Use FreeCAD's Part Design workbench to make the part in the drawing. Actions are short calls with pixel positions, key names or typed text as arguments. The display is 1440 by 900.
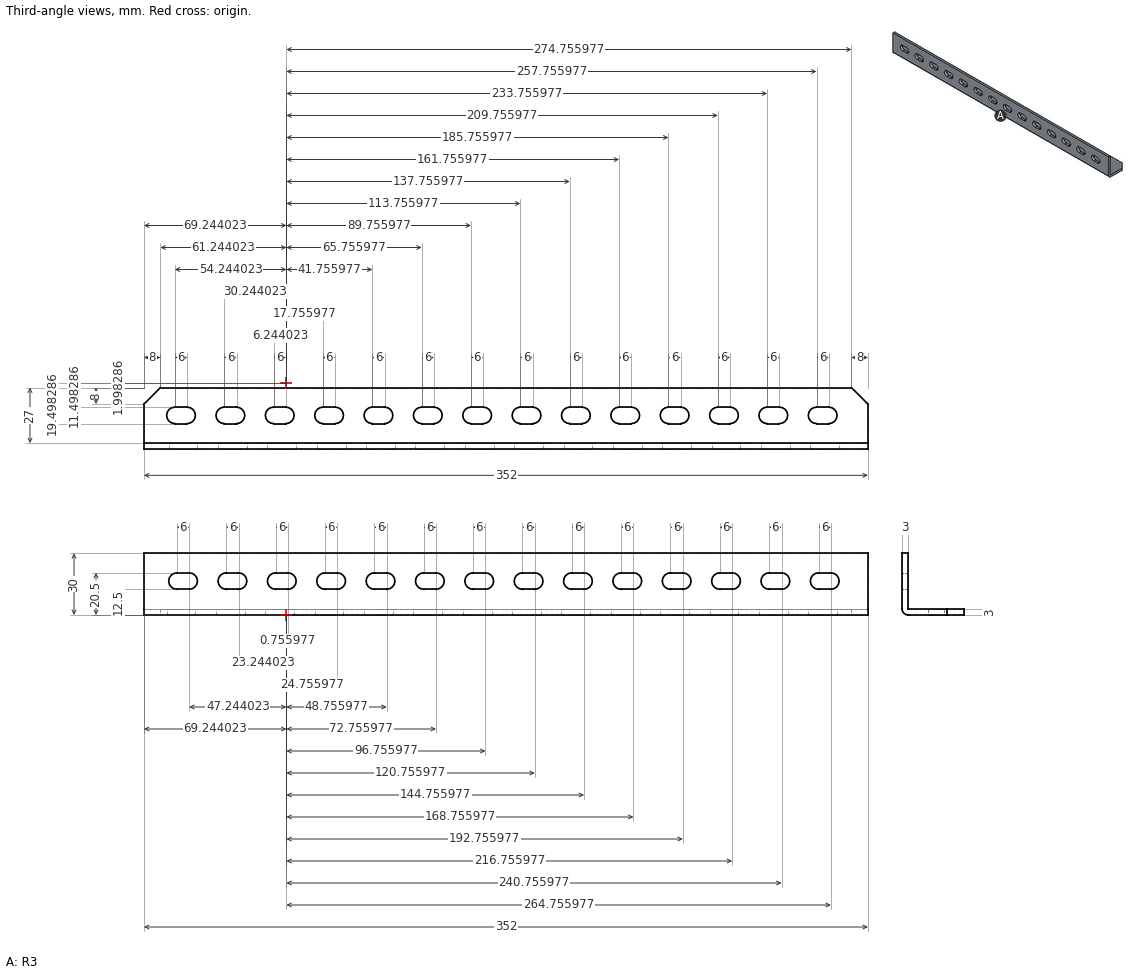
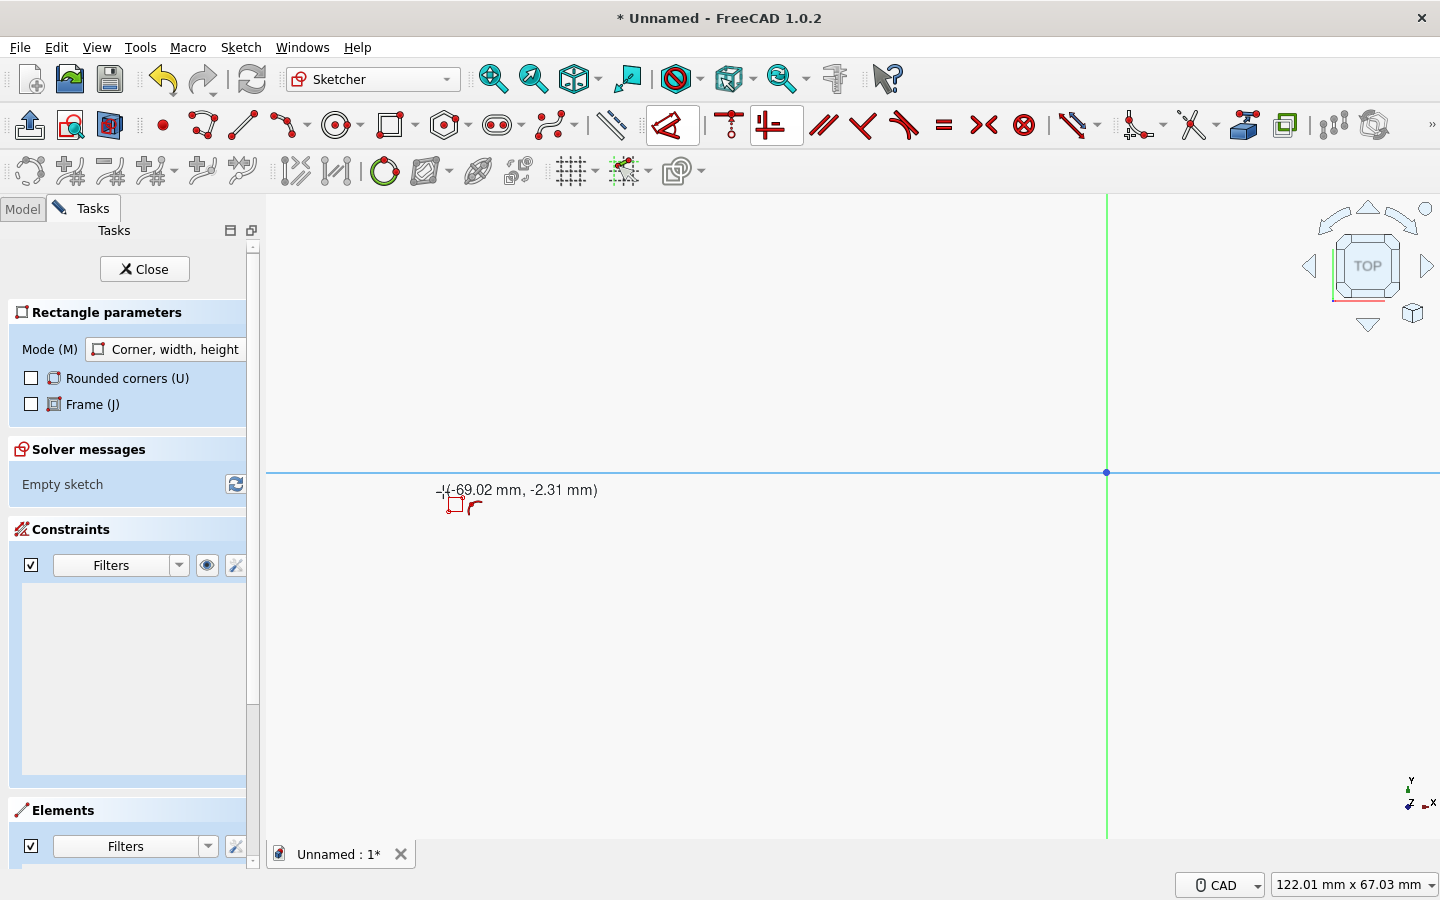
click(440, 492)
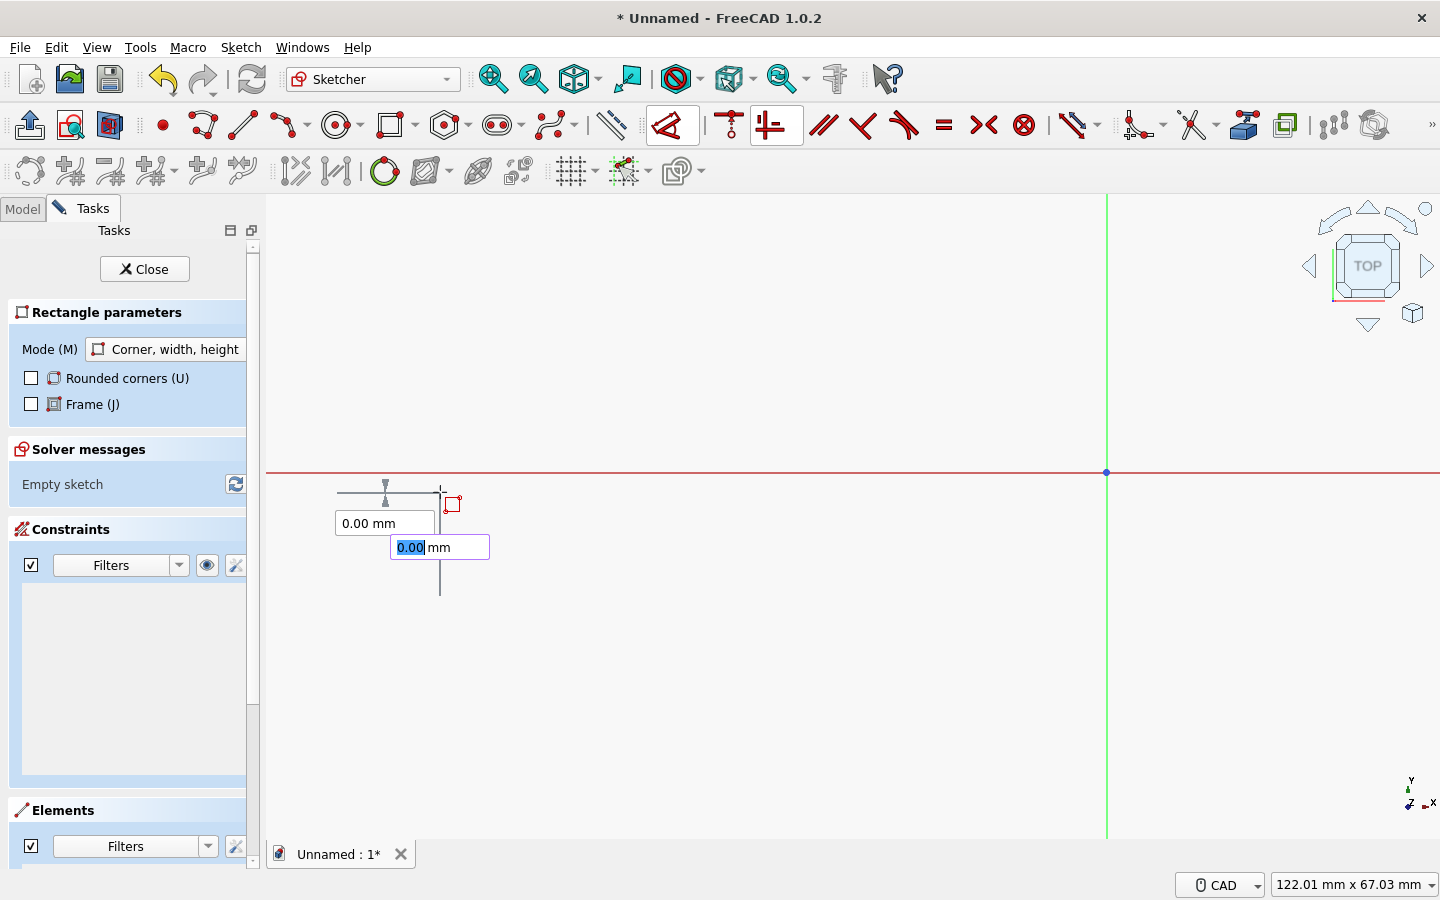
scroll(443, 492, down, 8)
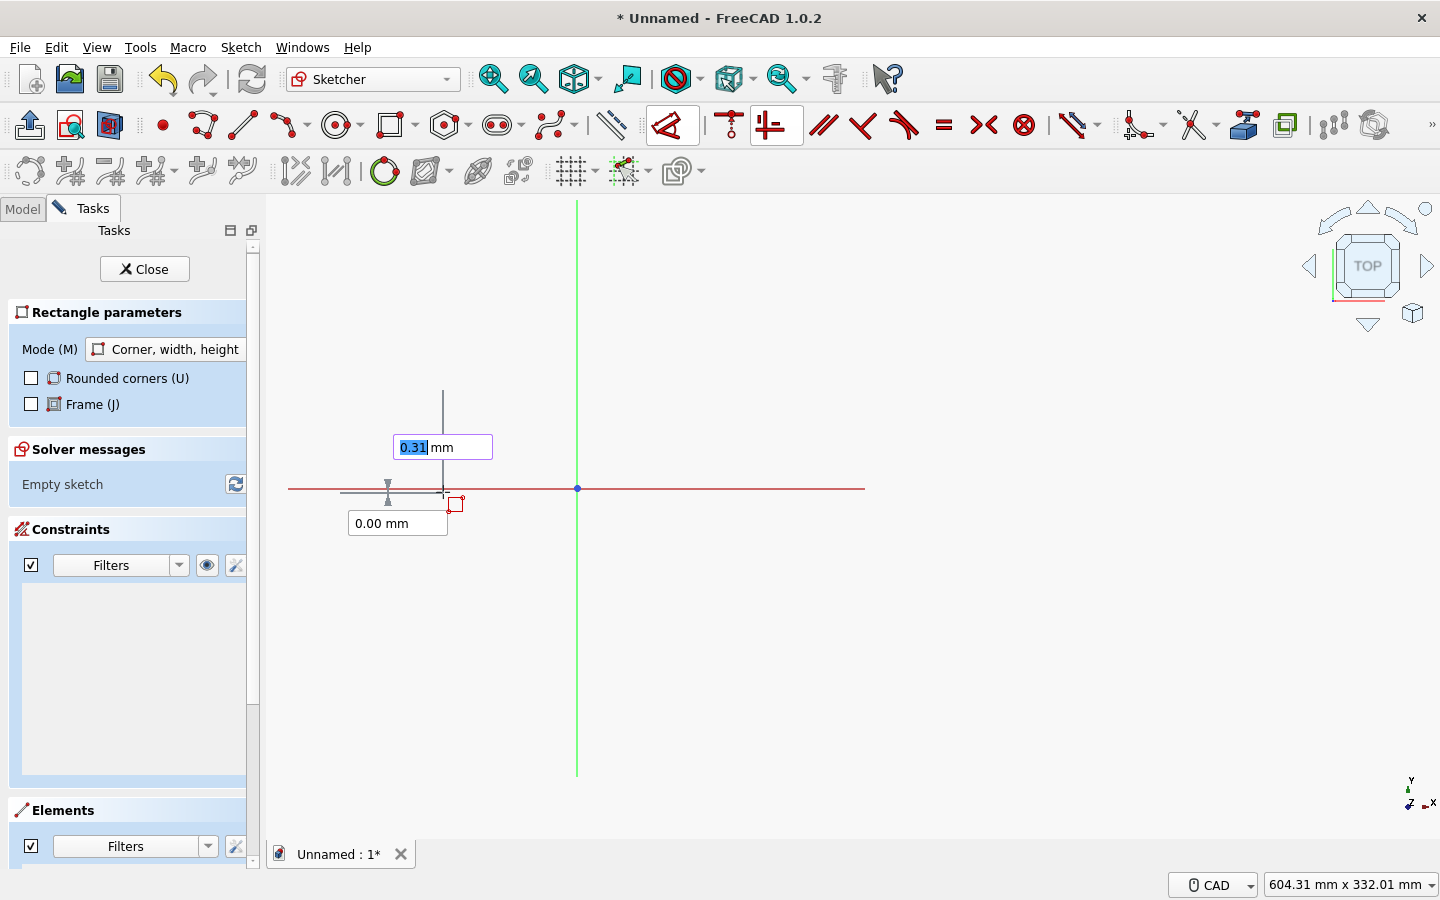
click(1126, 545)
key(Escape)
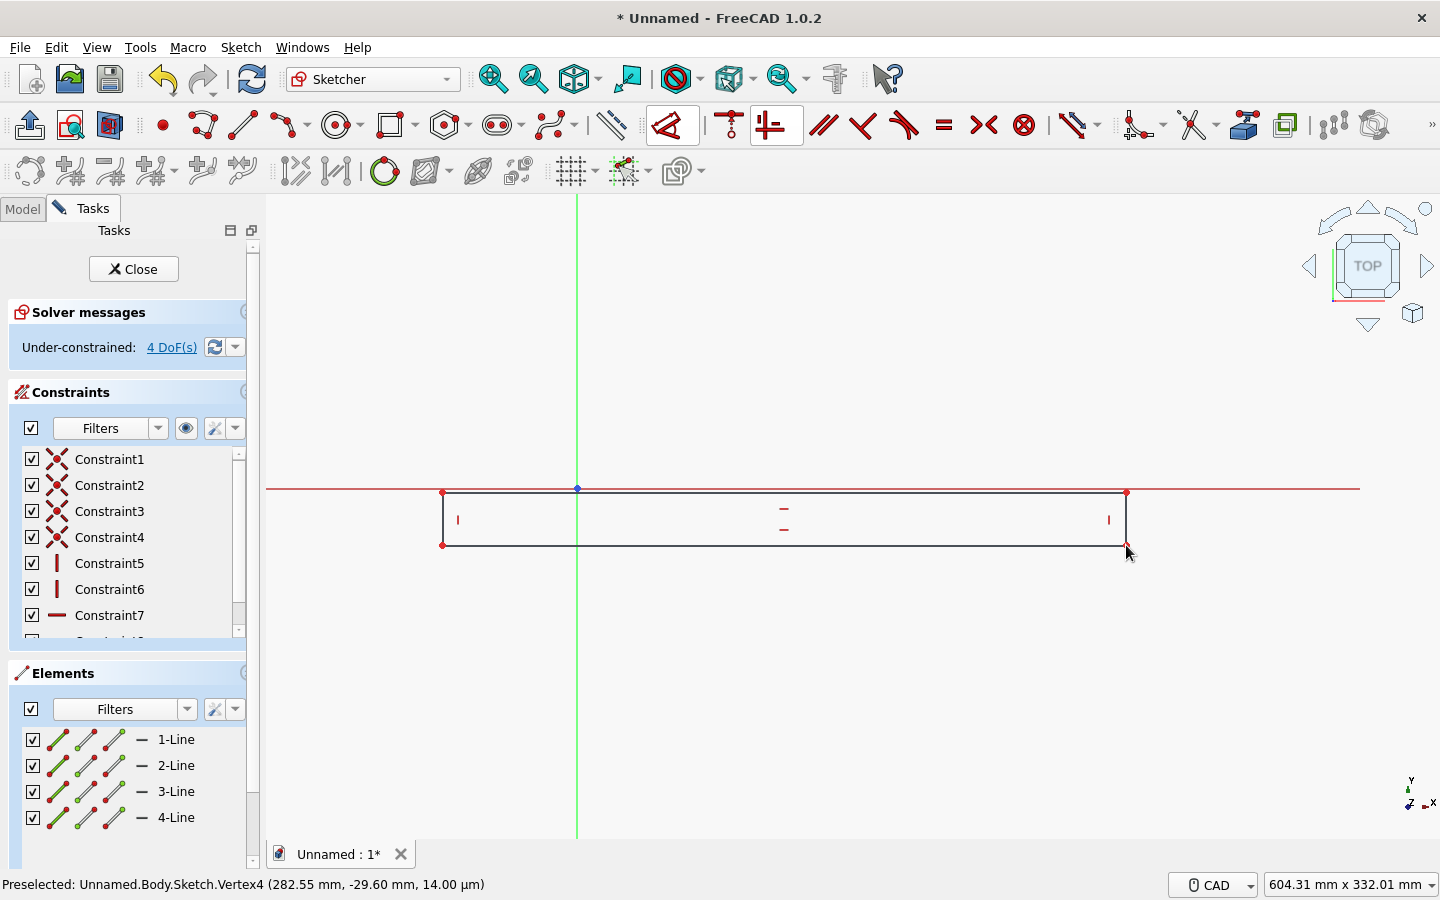
click(666, 126)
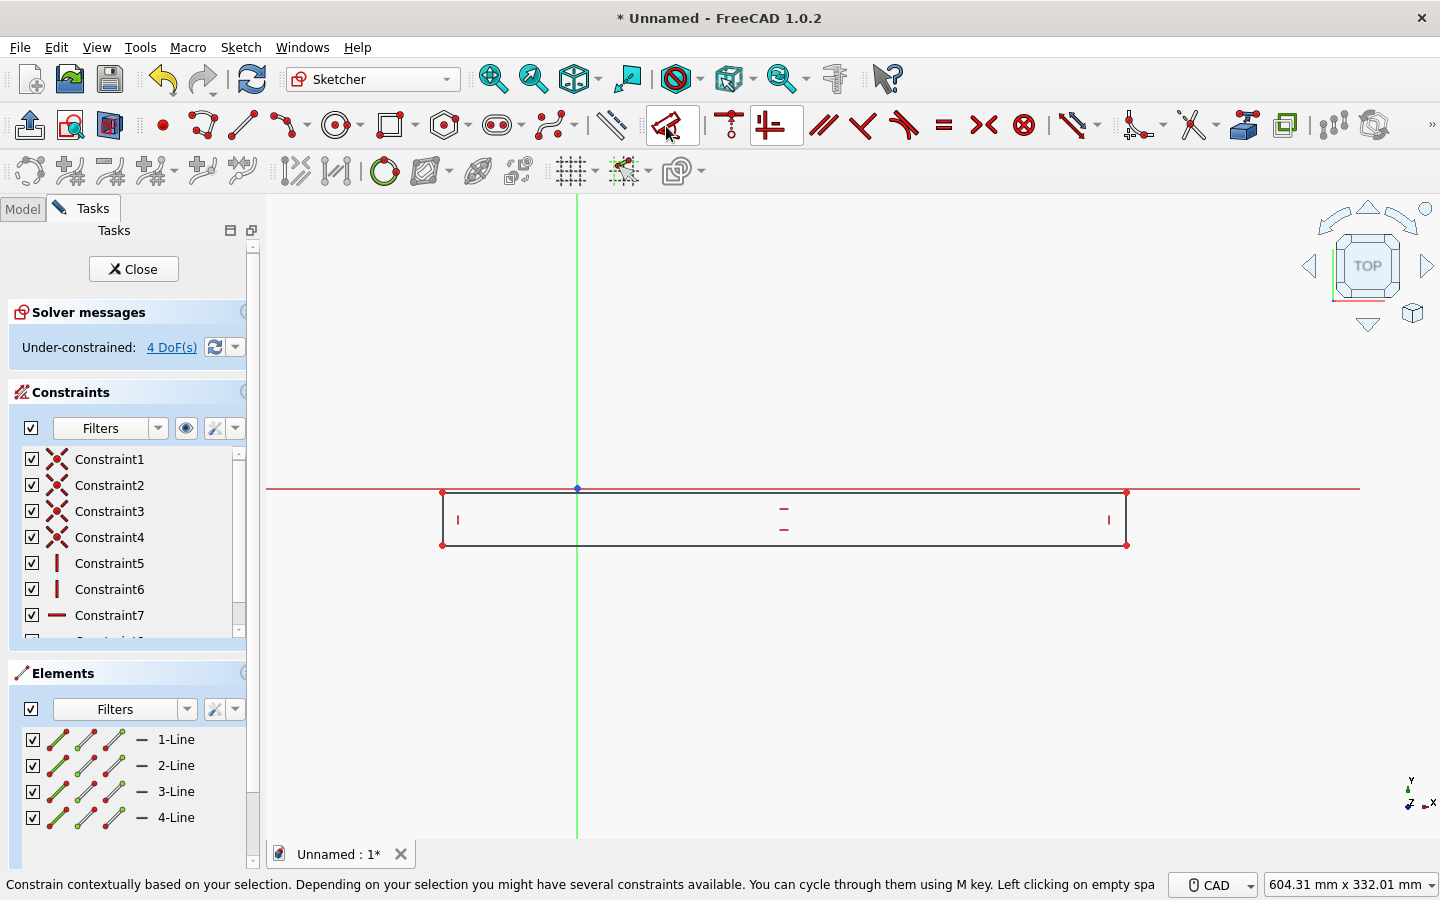
click(443, 509)
click(409, 519)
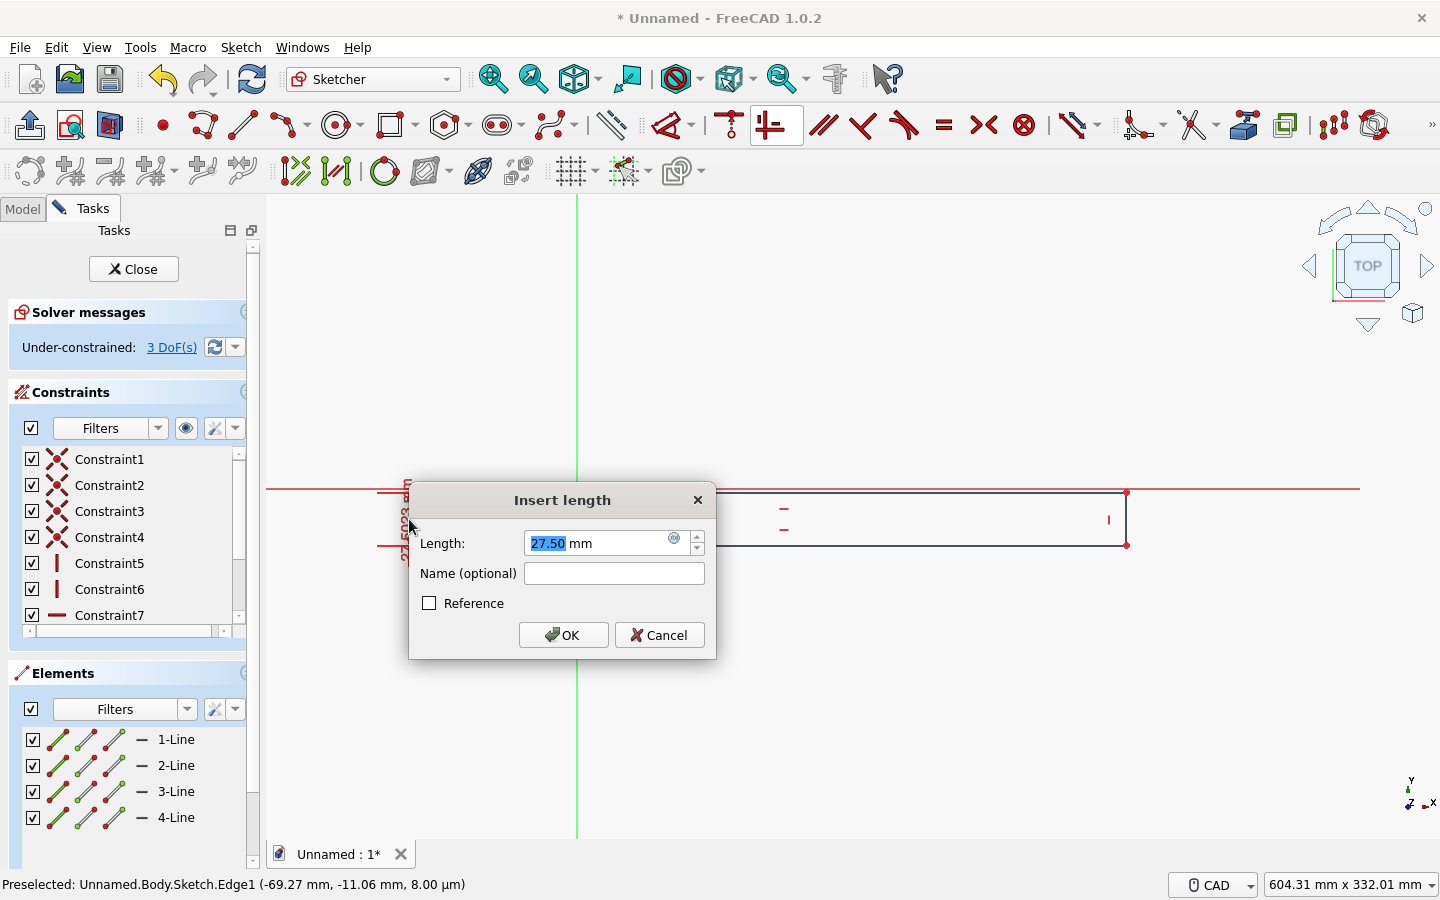
text(27)
key(Return)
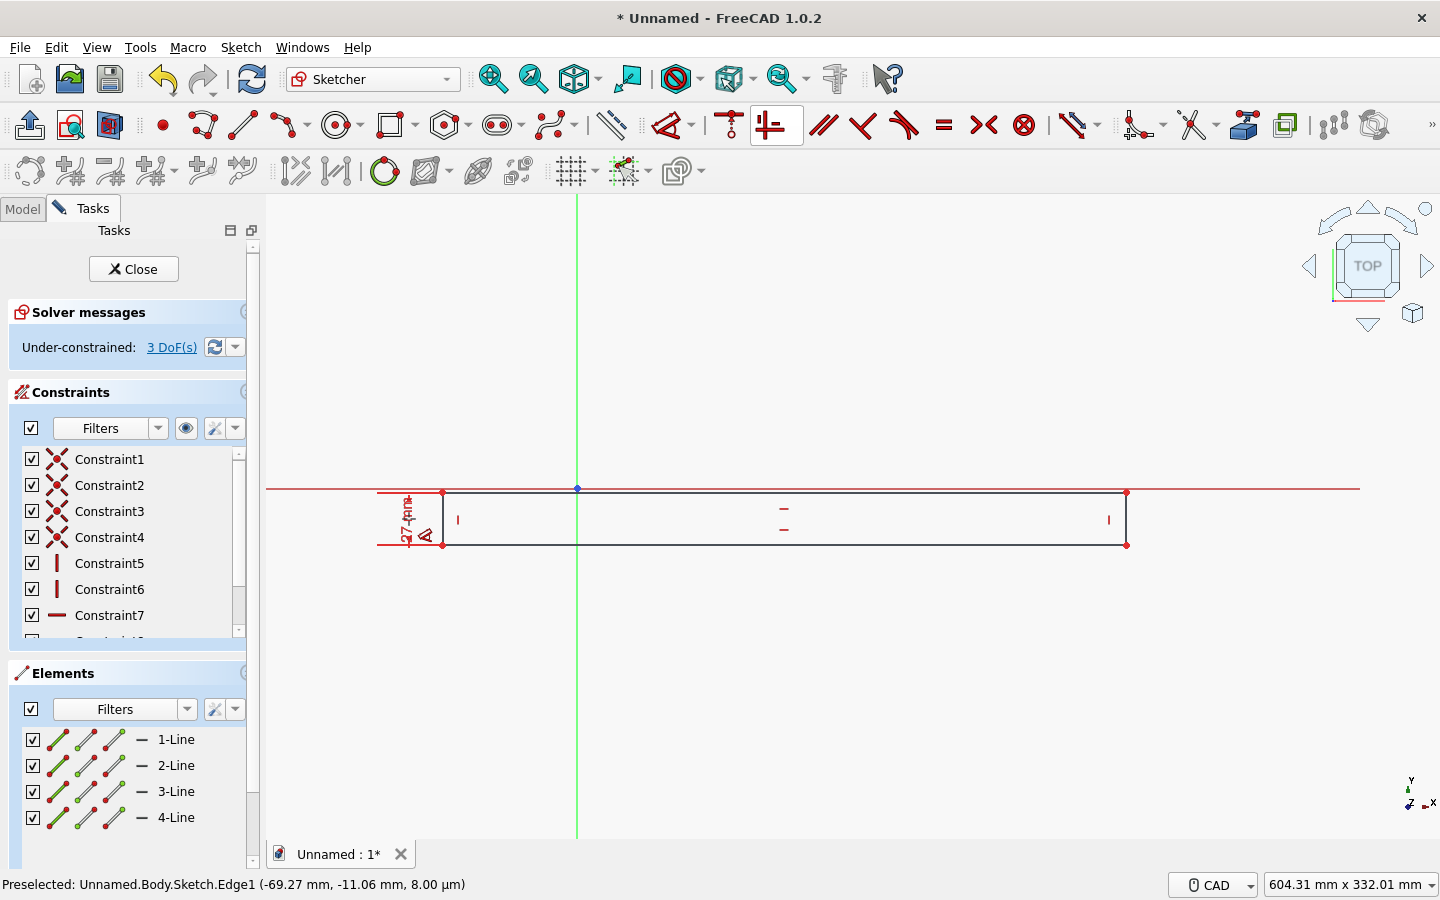
click(648, 545)
click(784, 579)